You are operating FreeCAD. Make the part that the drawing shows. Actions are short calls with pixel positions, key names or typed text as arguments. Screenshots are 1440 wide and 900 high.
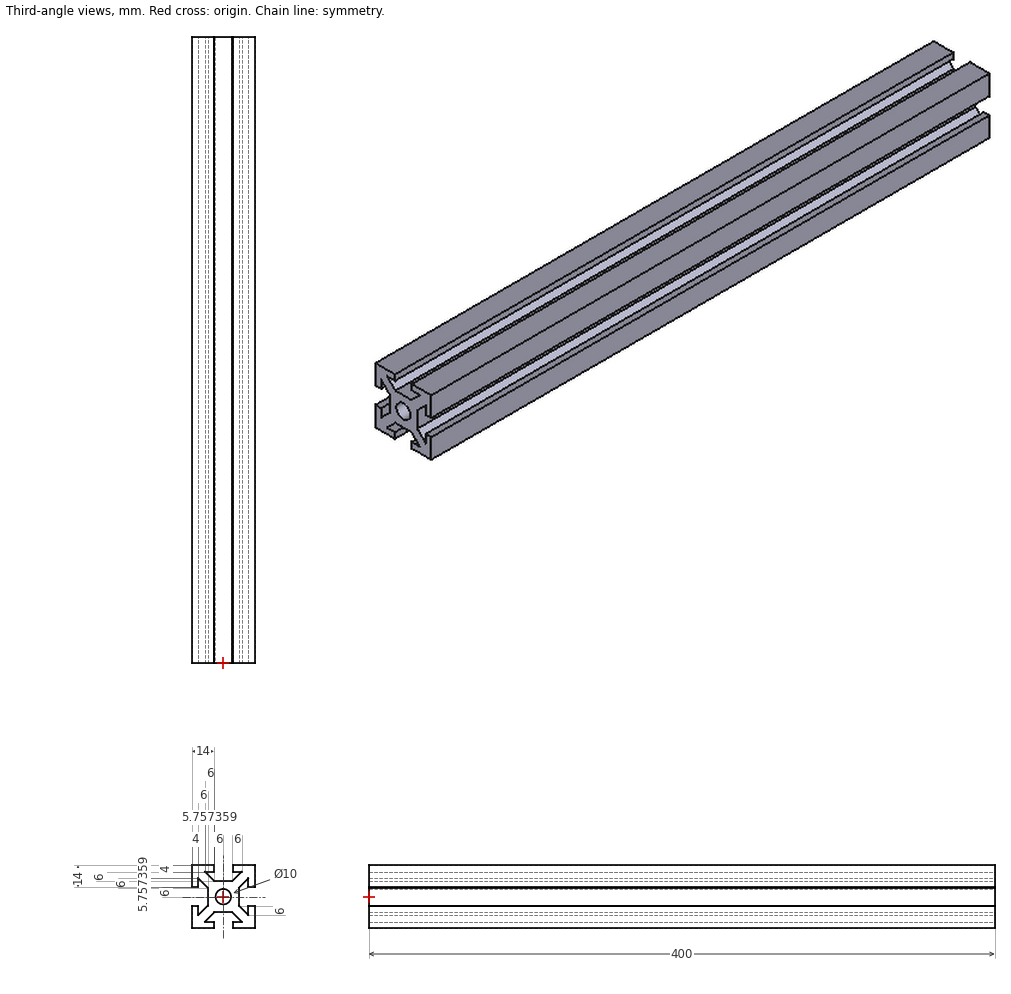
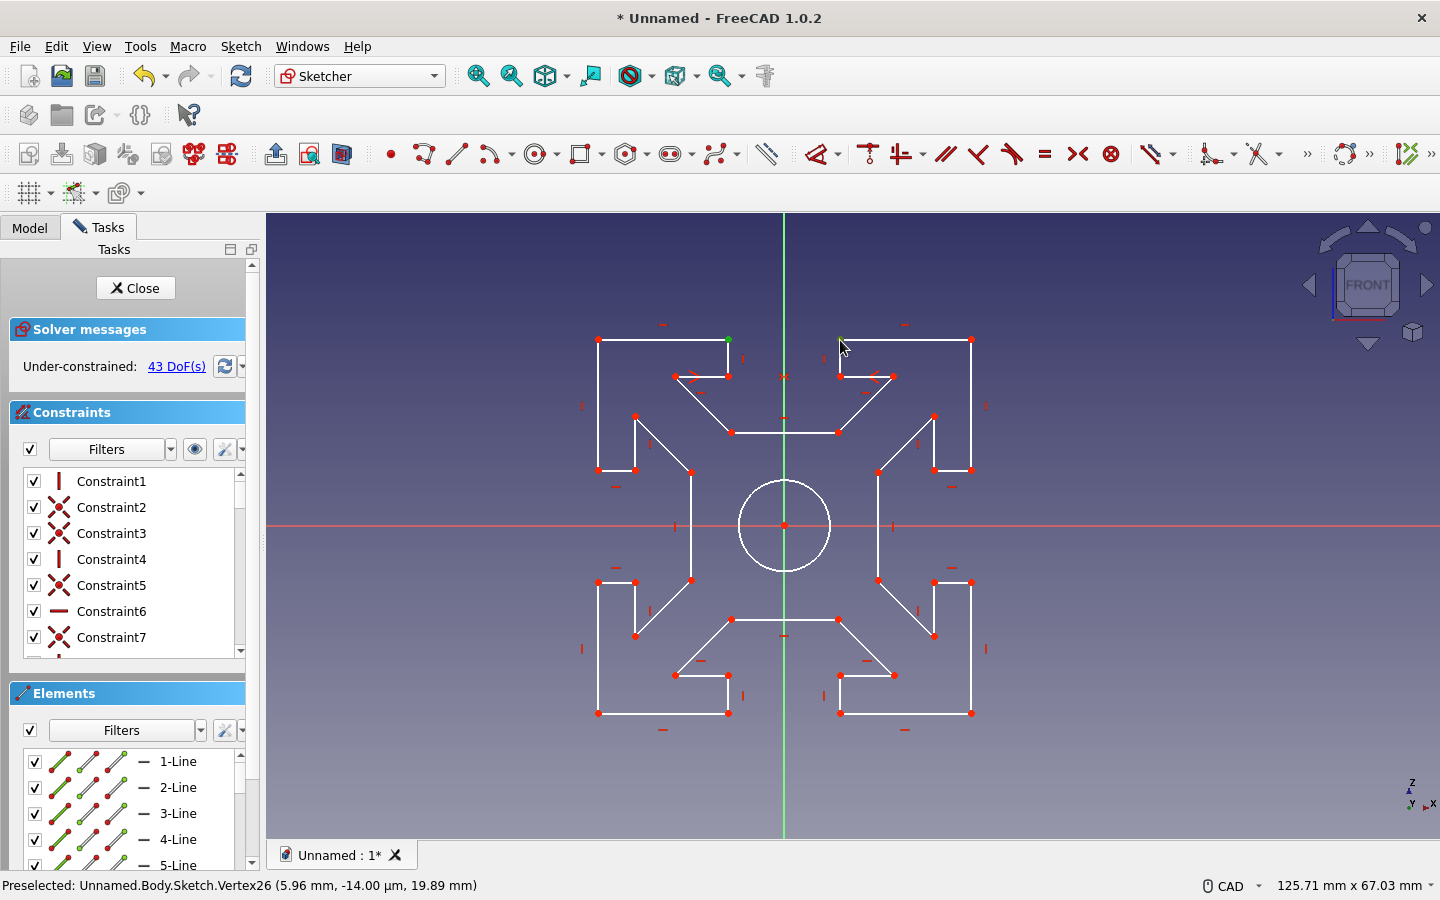
click(784, 770)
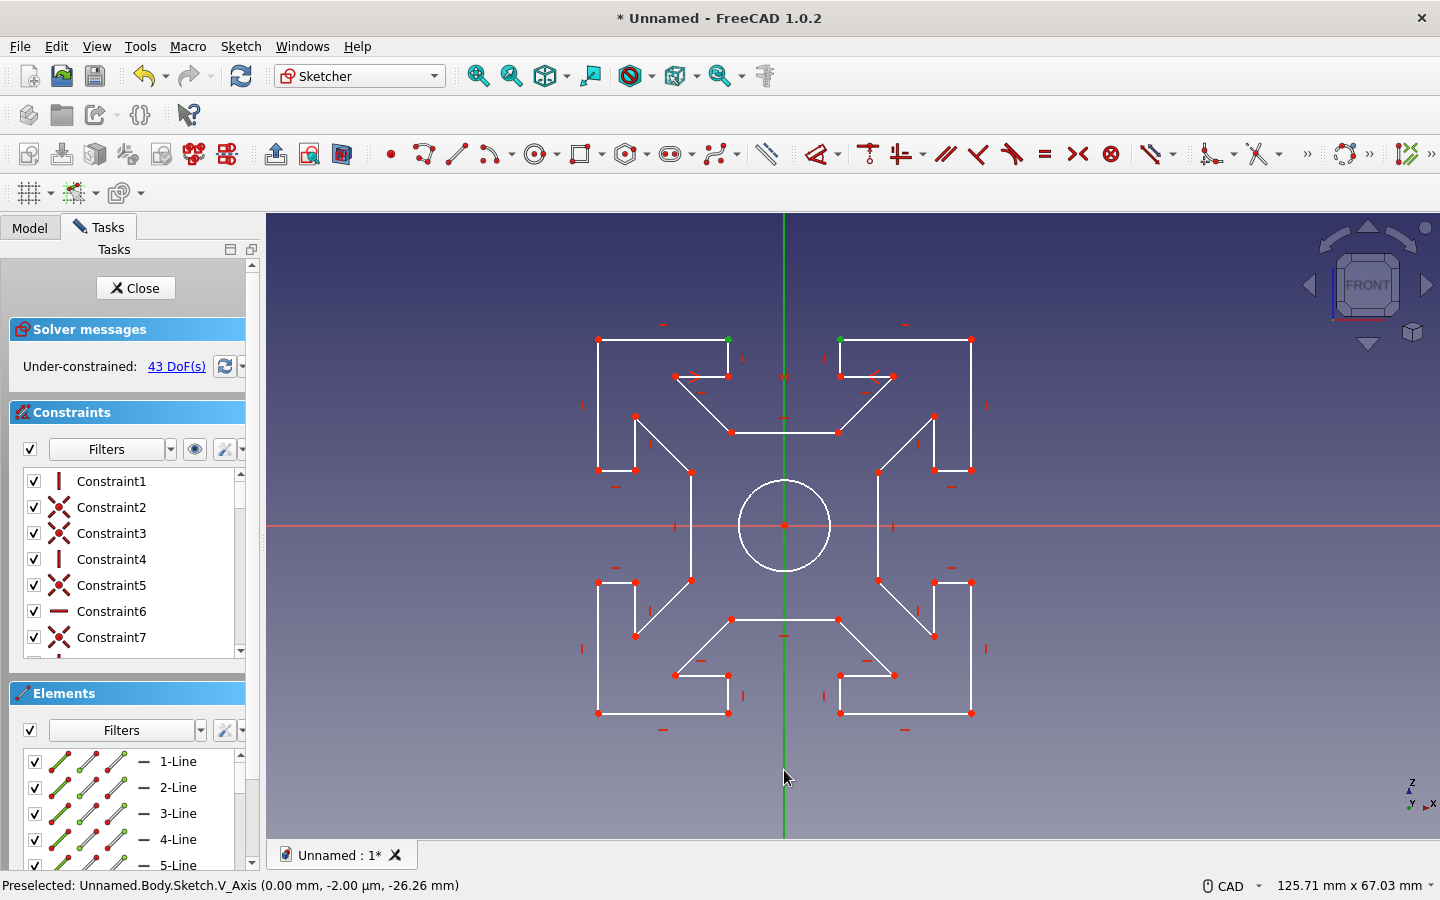
key(s)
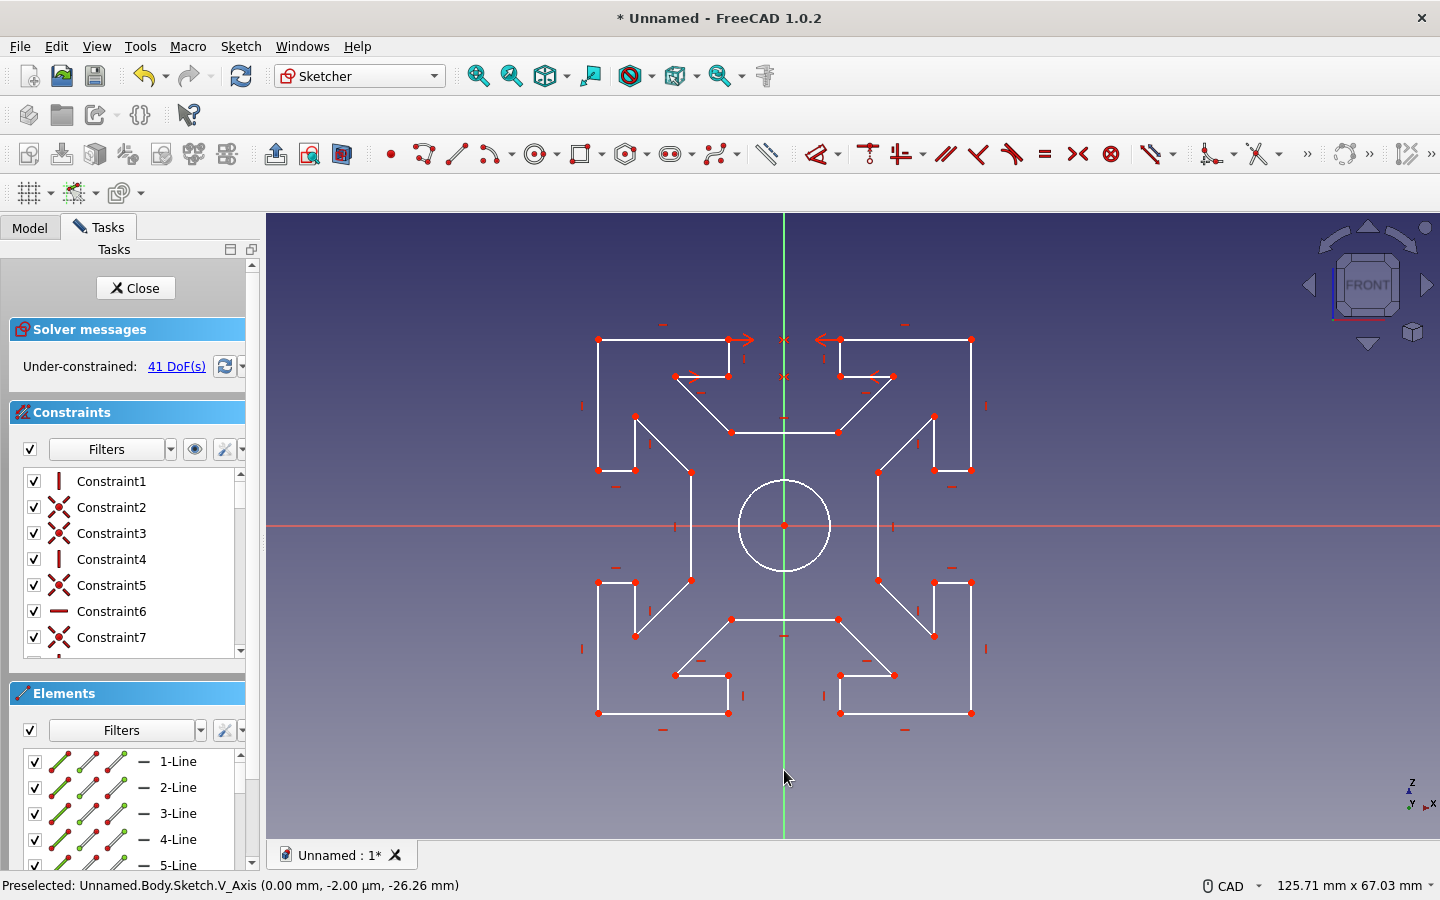
click(598, 471)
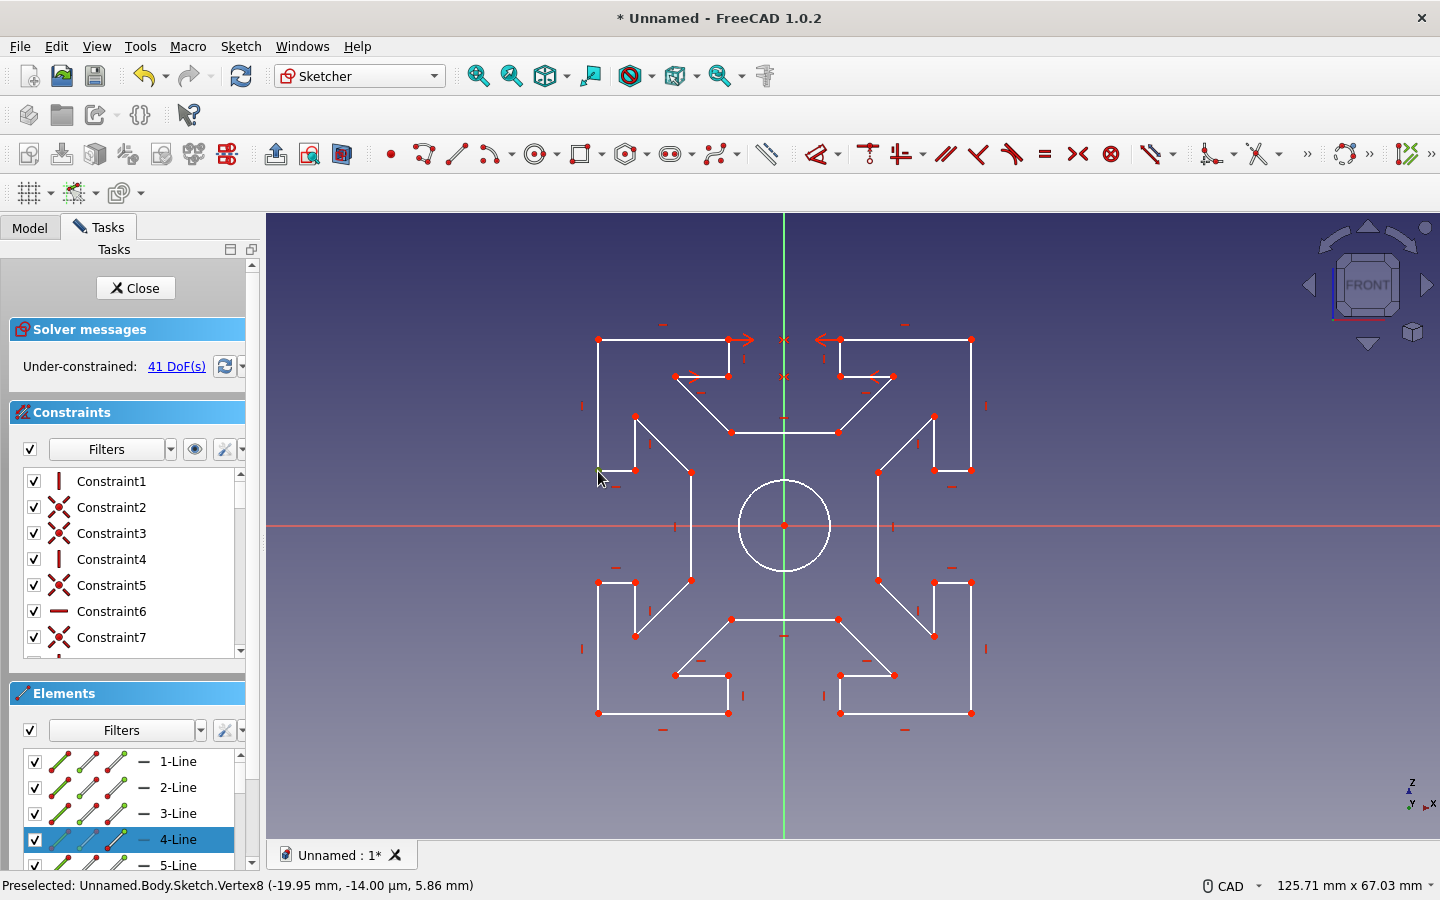
click(971, 471)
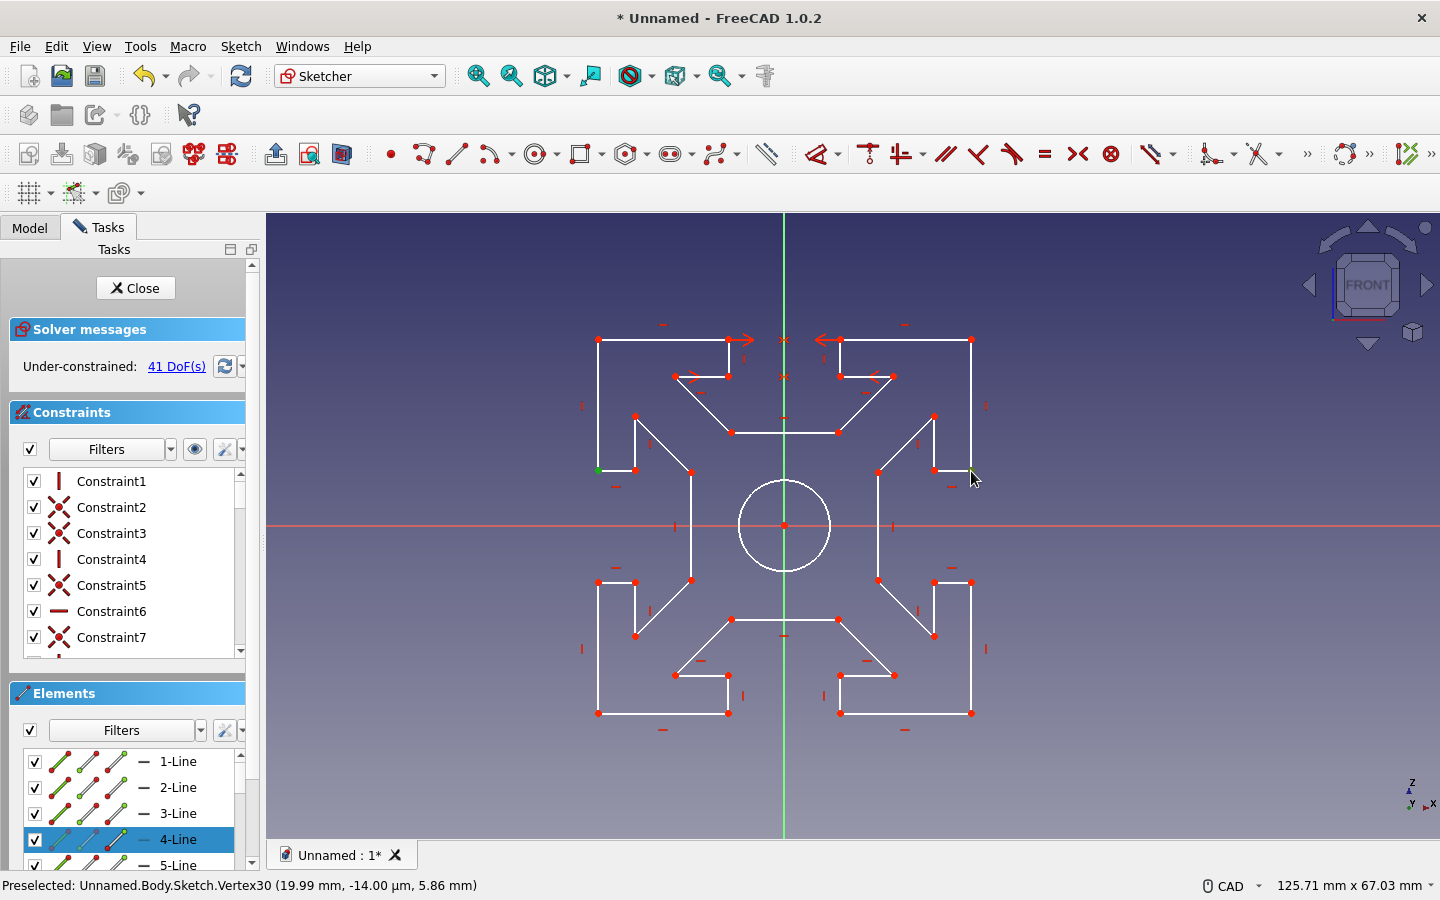
click(784, 770)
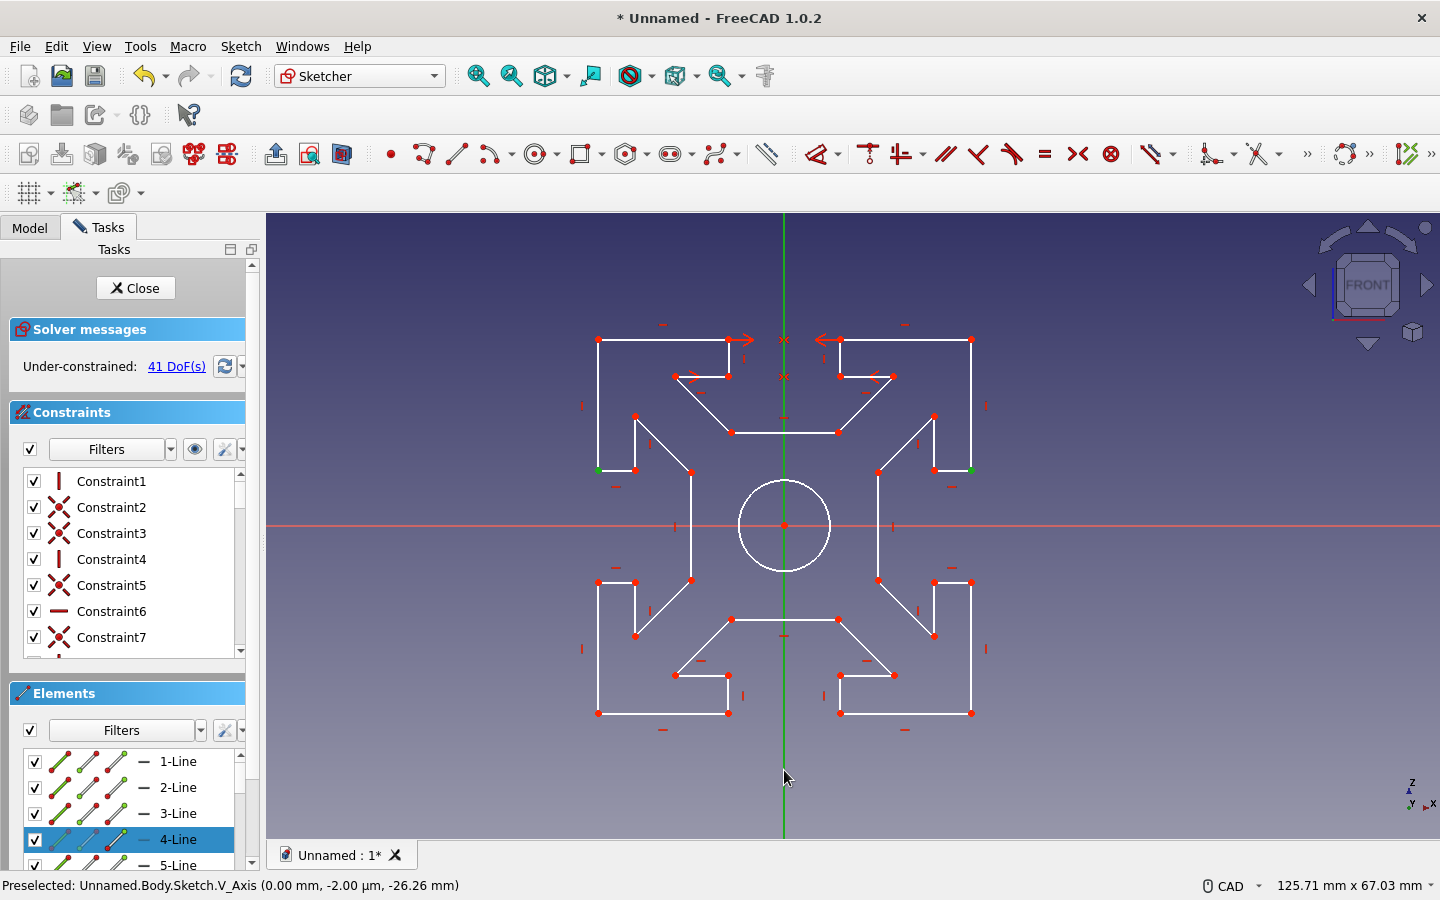
key(s)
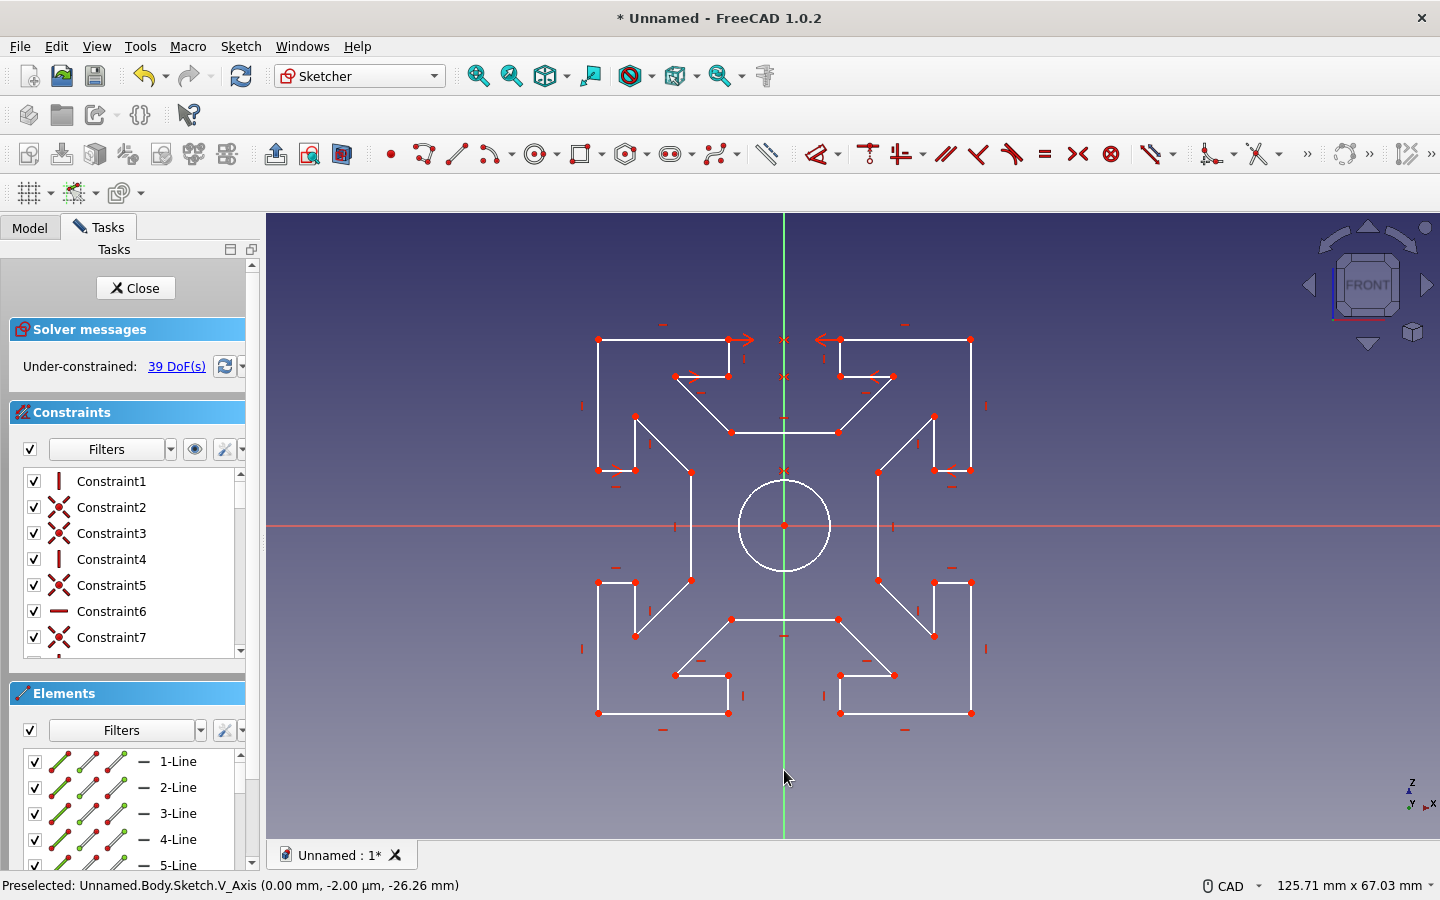
click(635, 417)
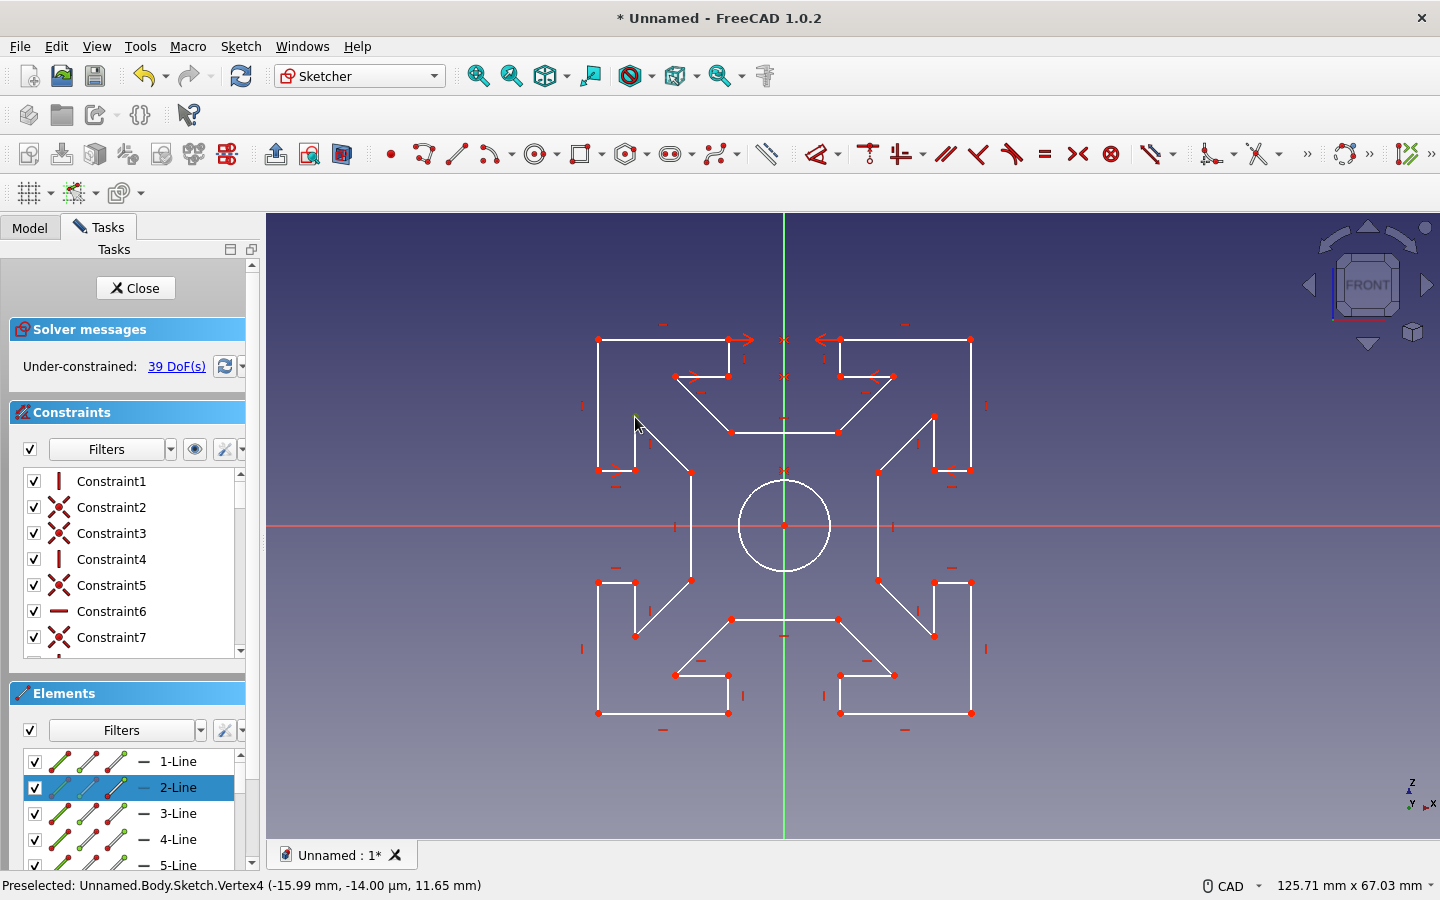
click(934, 417)